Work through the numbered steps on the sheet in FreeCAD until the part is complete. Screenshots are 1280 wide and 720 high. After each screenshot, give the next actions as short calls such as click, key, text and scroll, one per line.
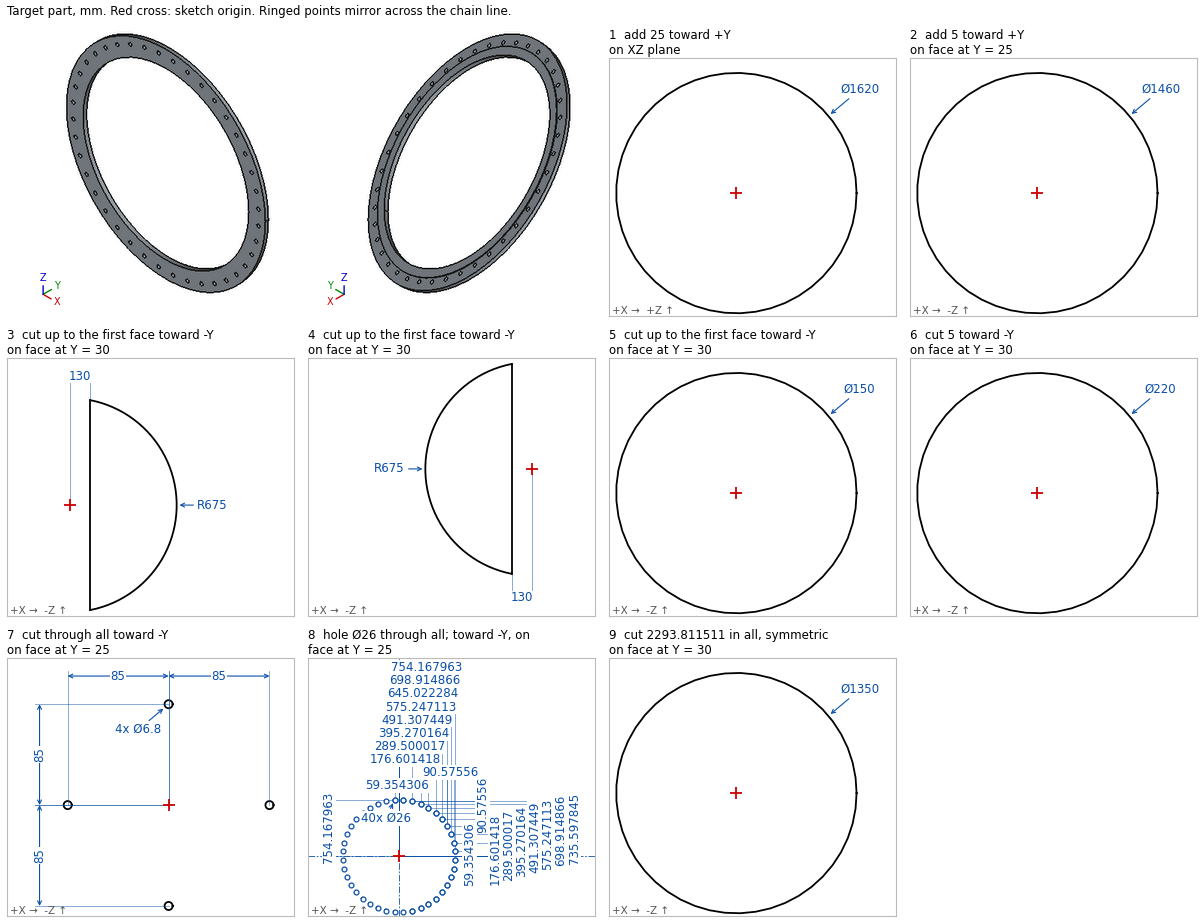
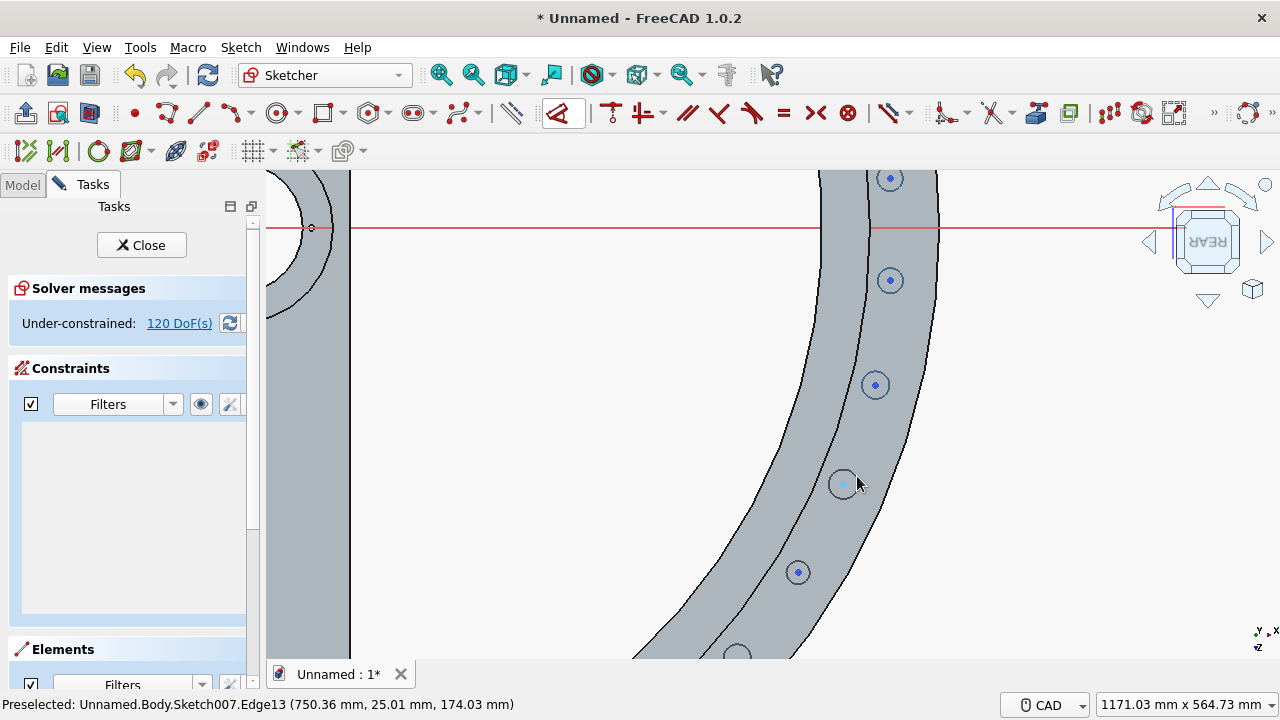
click(854, 474)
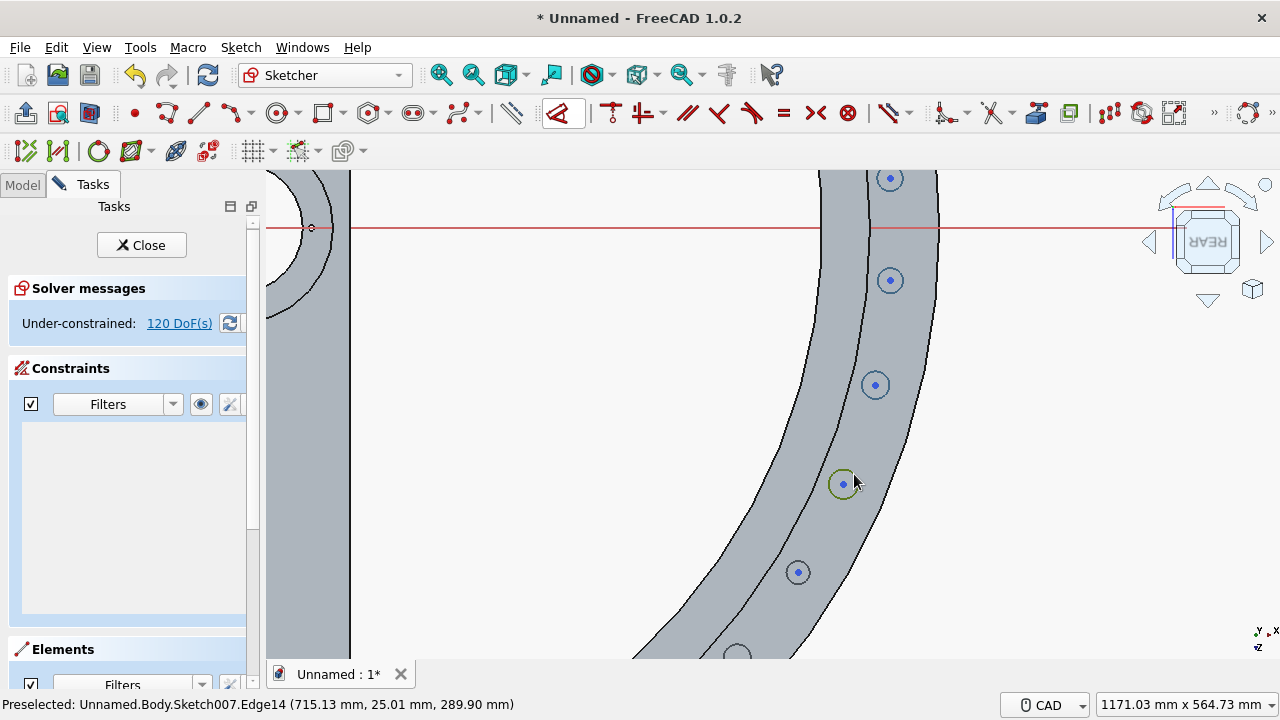
click(806, 564)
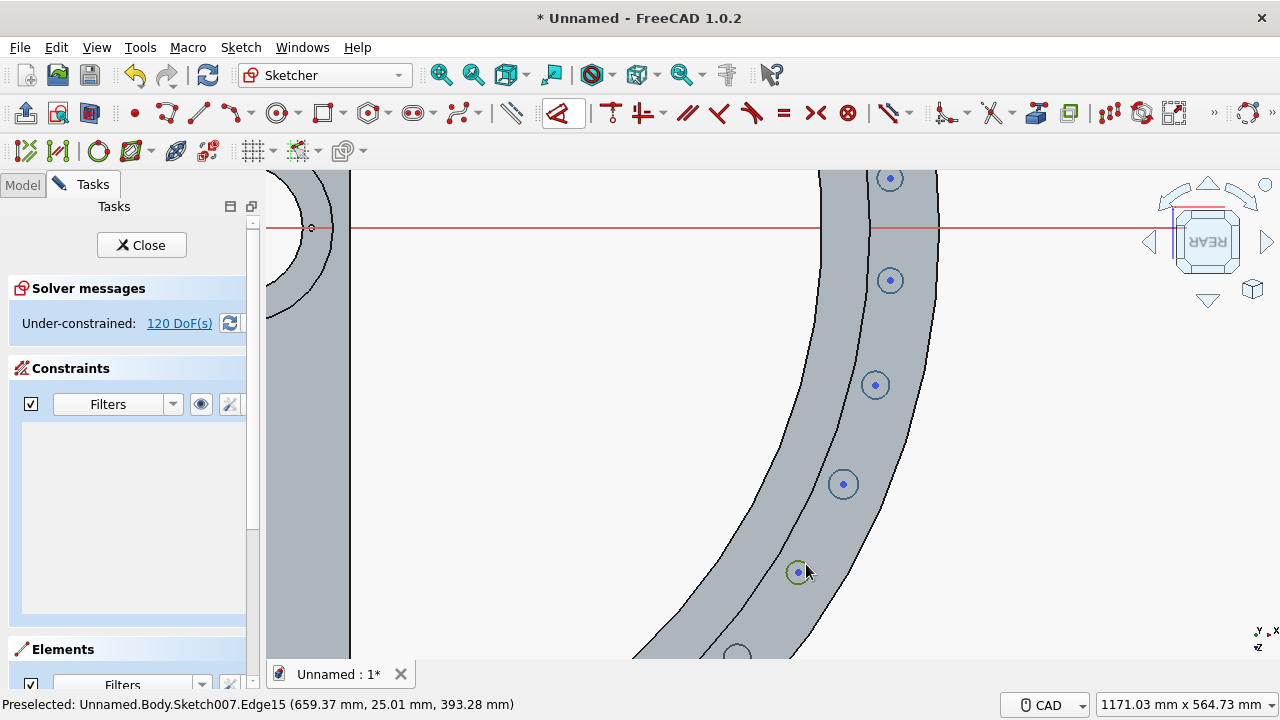
scroll(857, 476, down, 7)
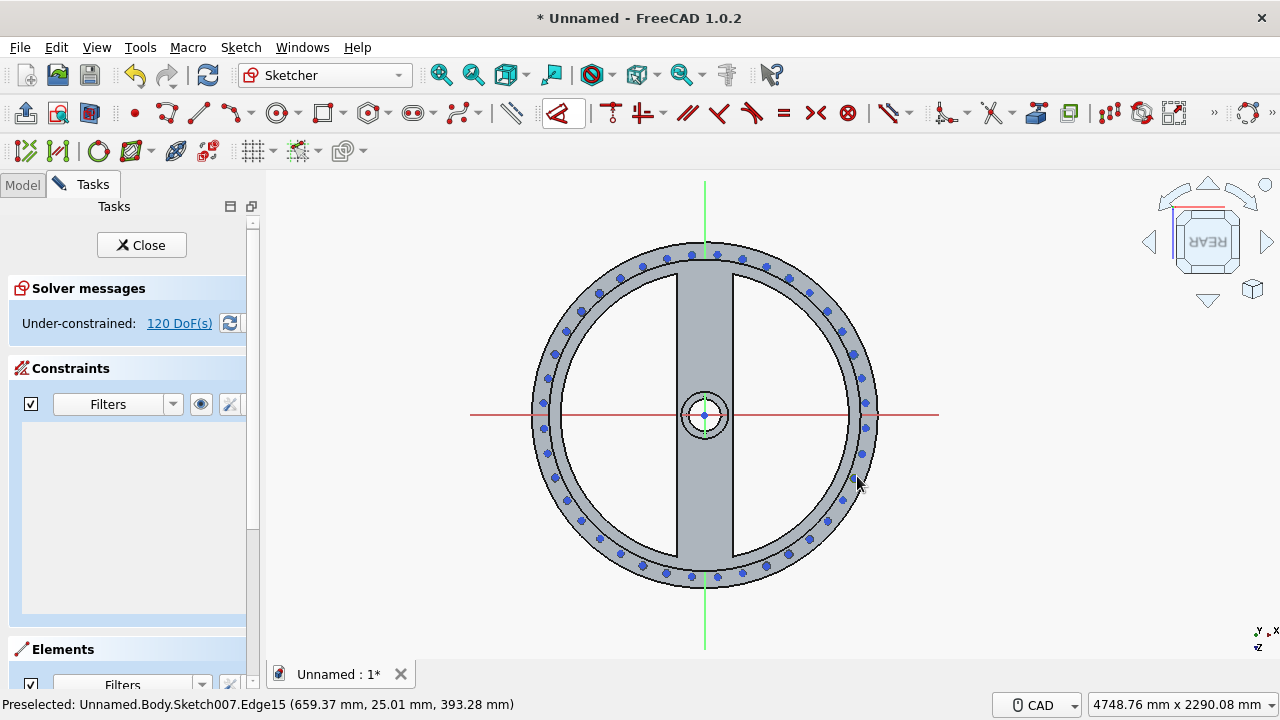
scroll(830, 519, up, 8)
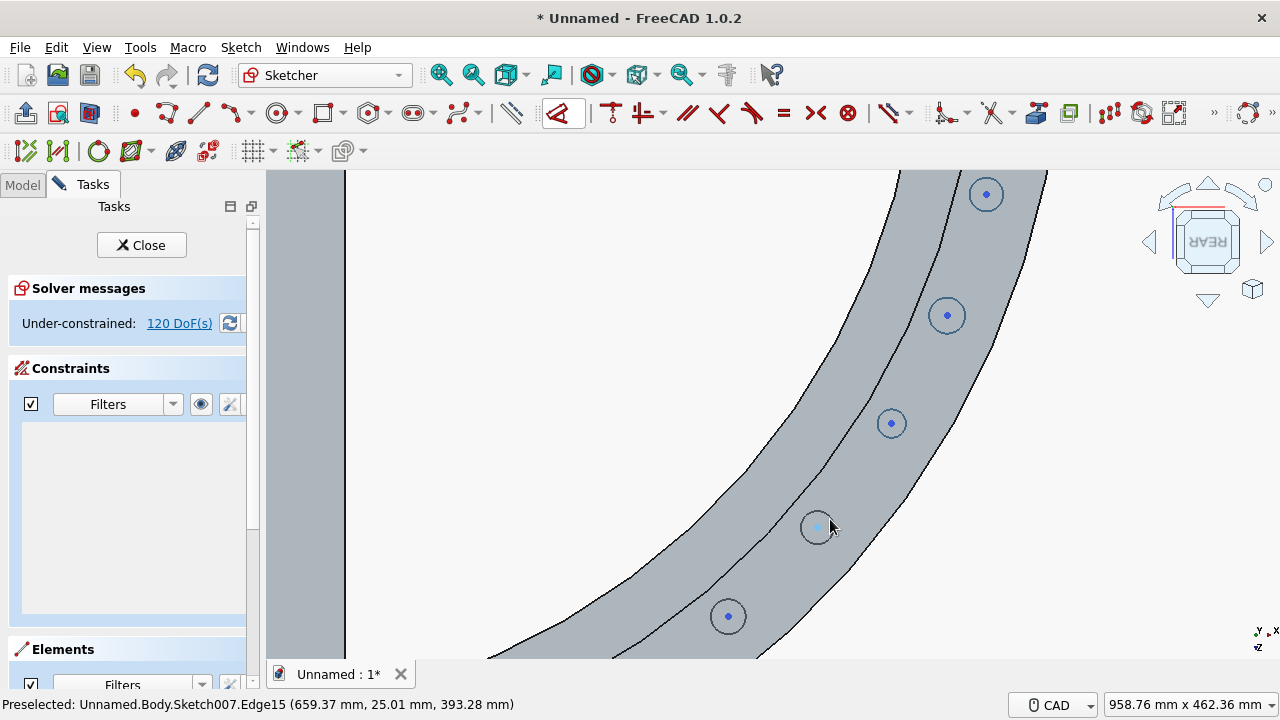
click(829, 516)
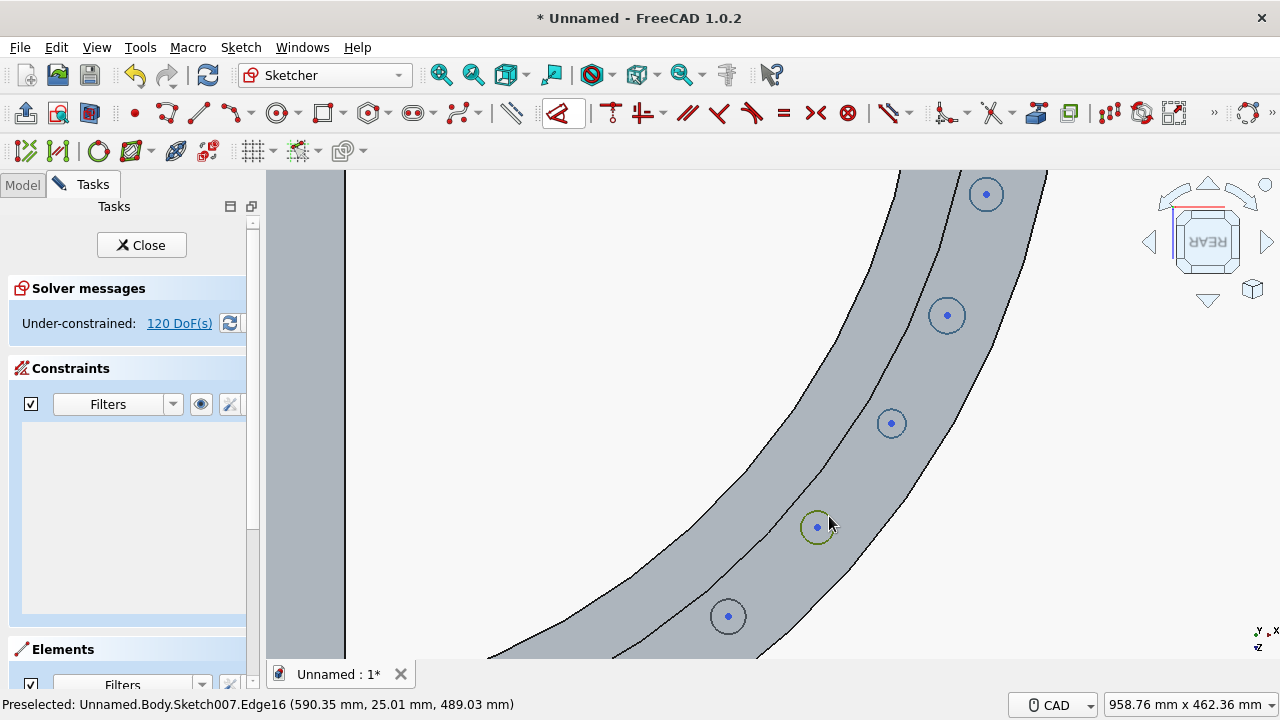
click(741, 604)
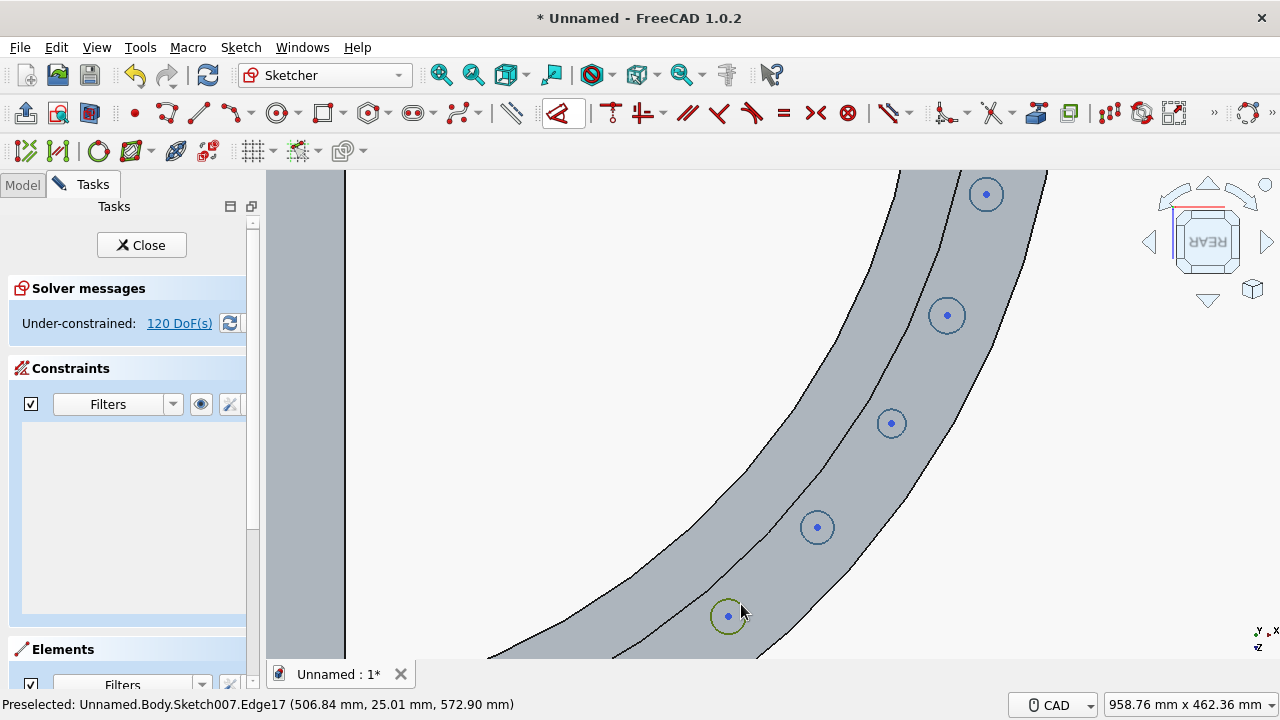
scroll(830, 519, down, 8)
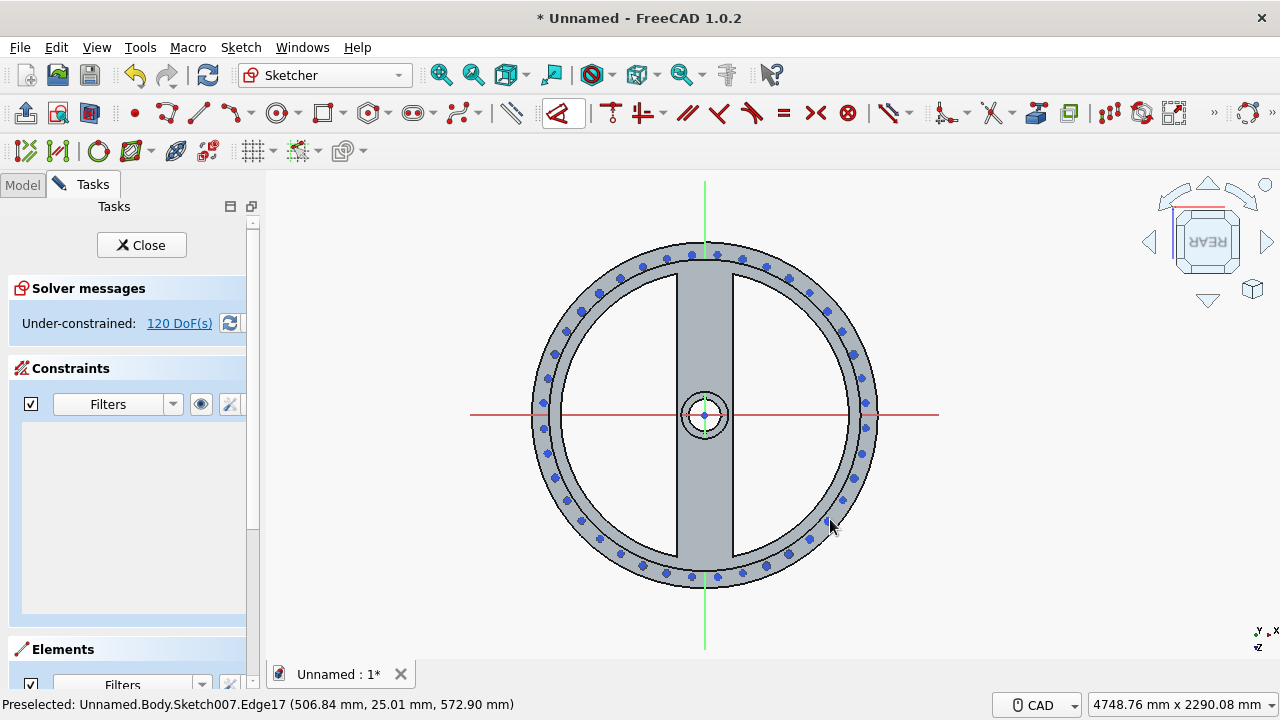
scroll(792, 552, up, 7)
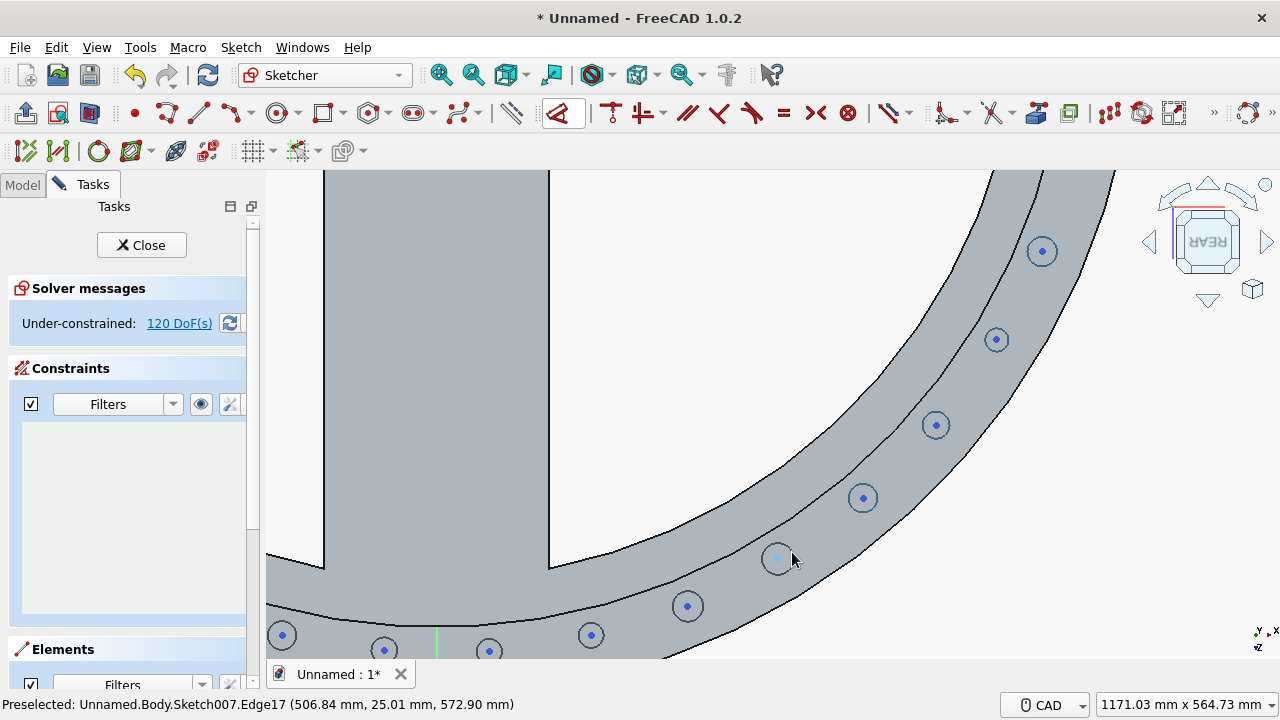
click(789, 548)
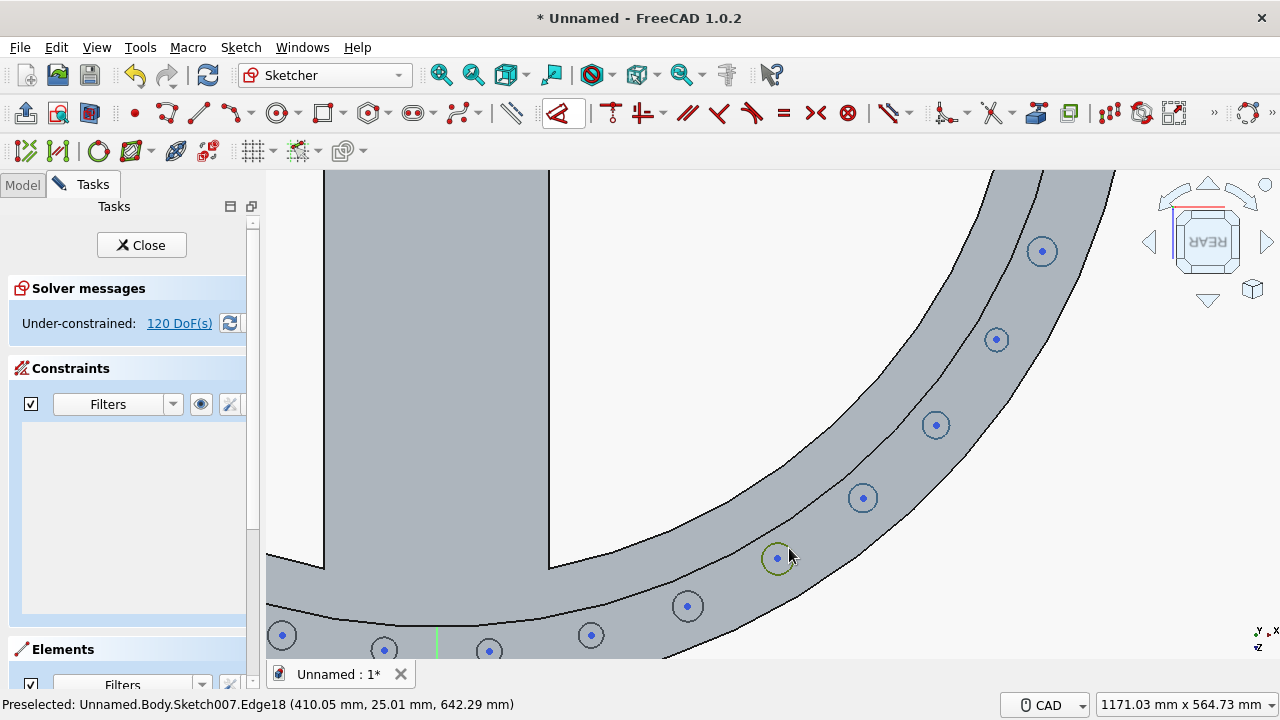
click(699, 596)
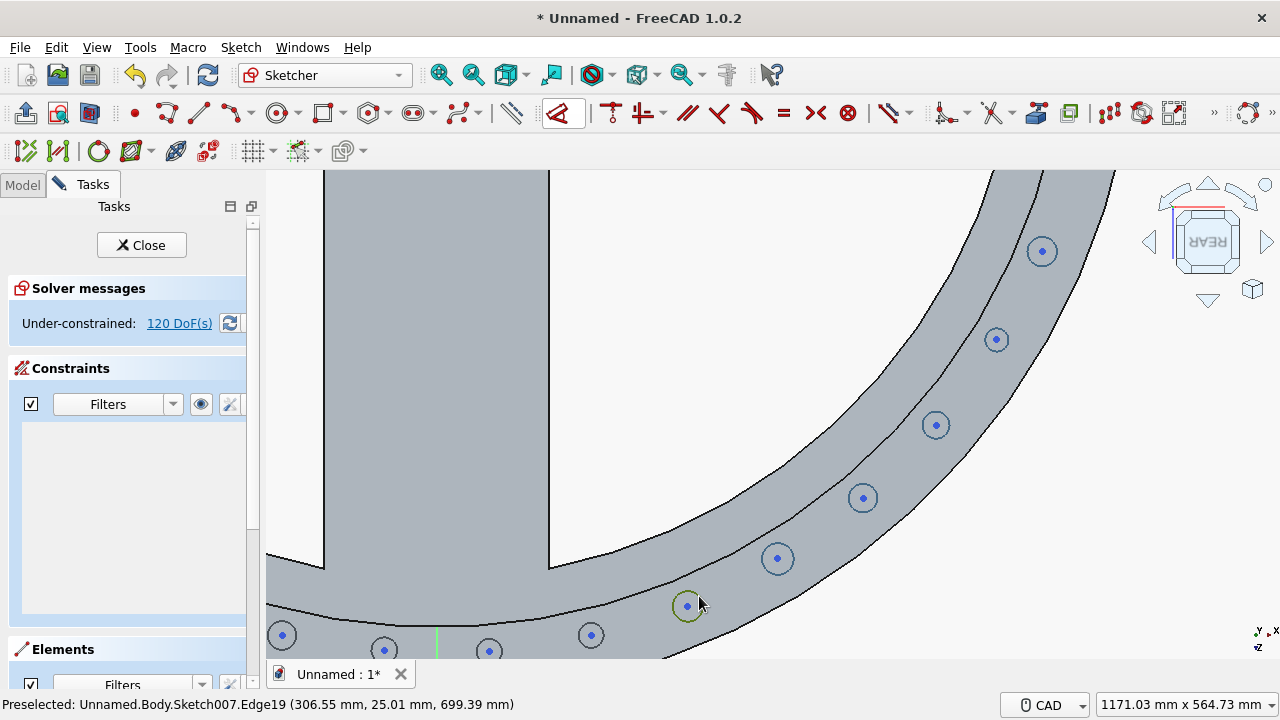
click(600, 627)